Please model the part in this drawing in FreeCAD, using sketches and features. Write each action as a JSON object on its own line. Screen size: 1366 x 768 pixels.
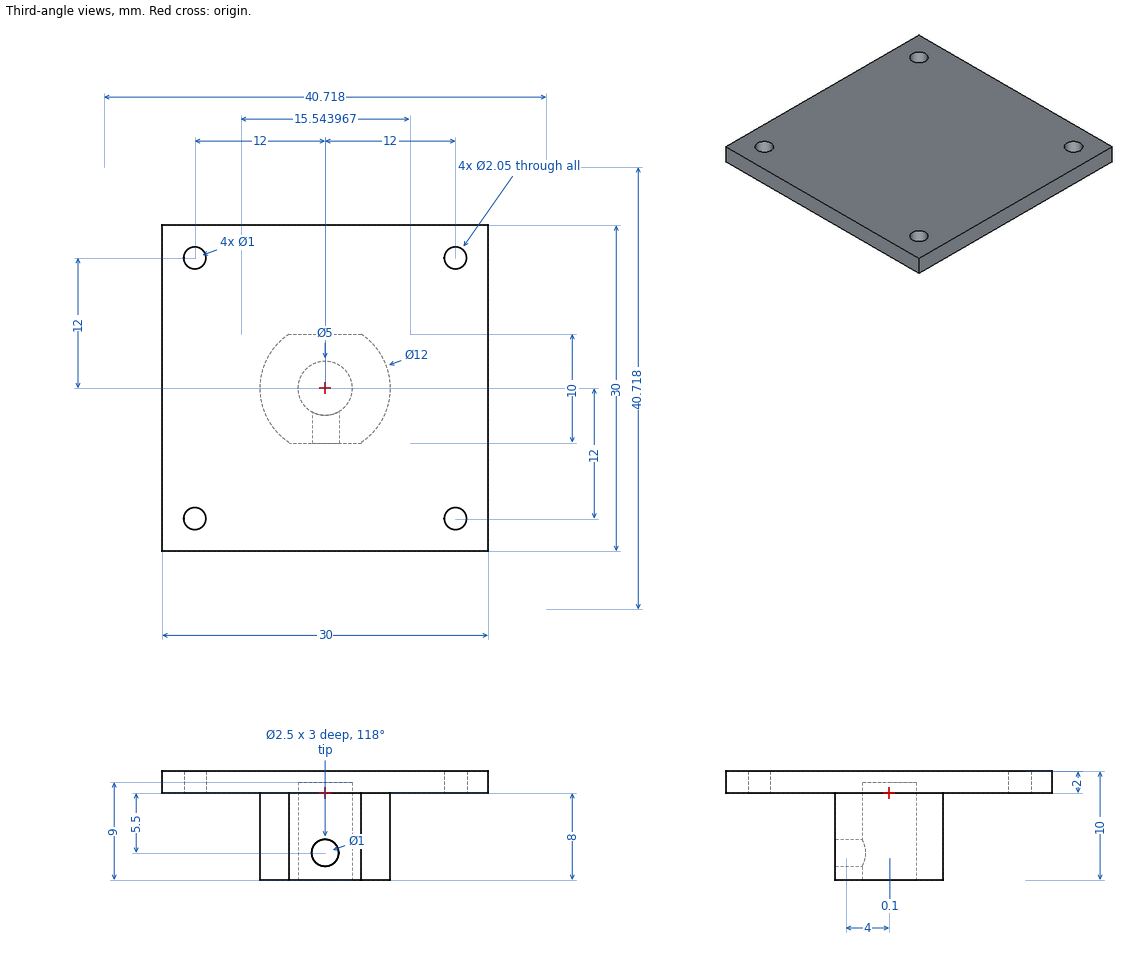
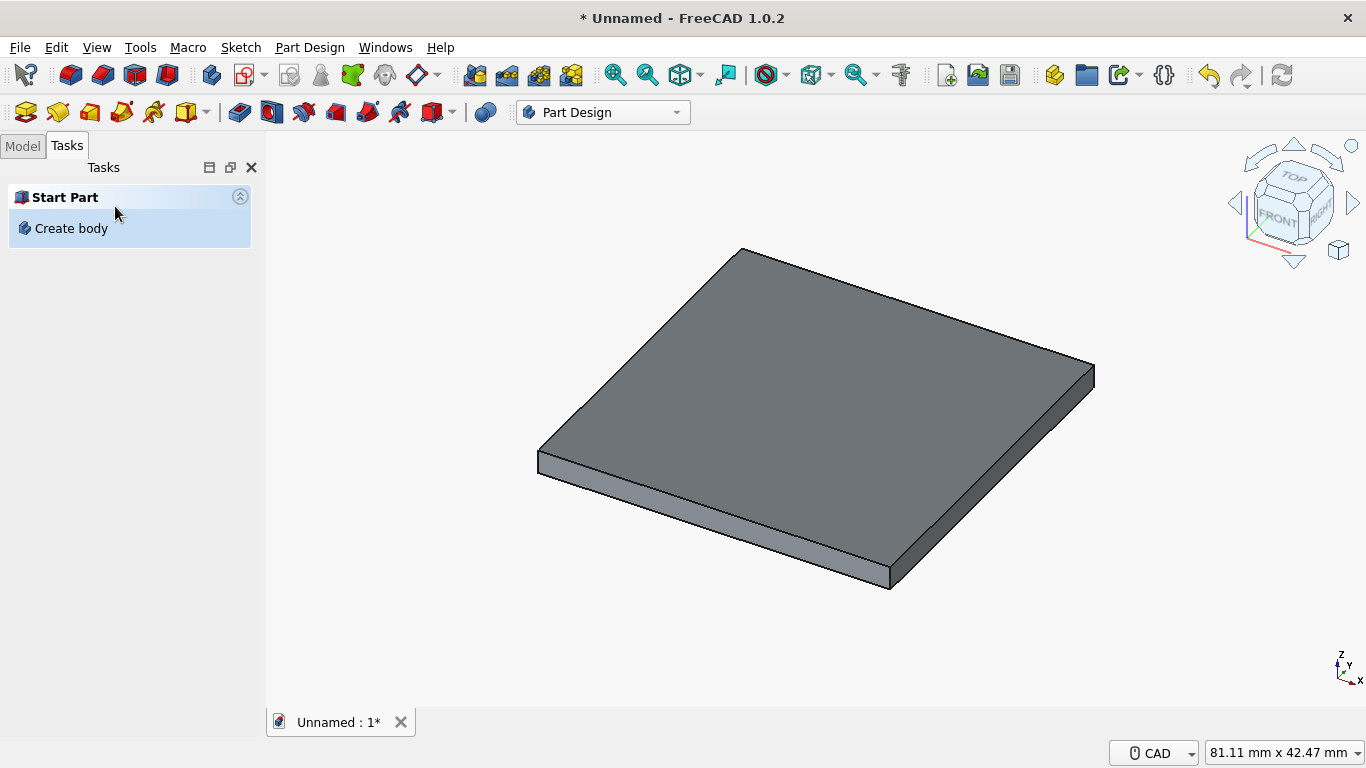
{"action": "key", "text": "5"}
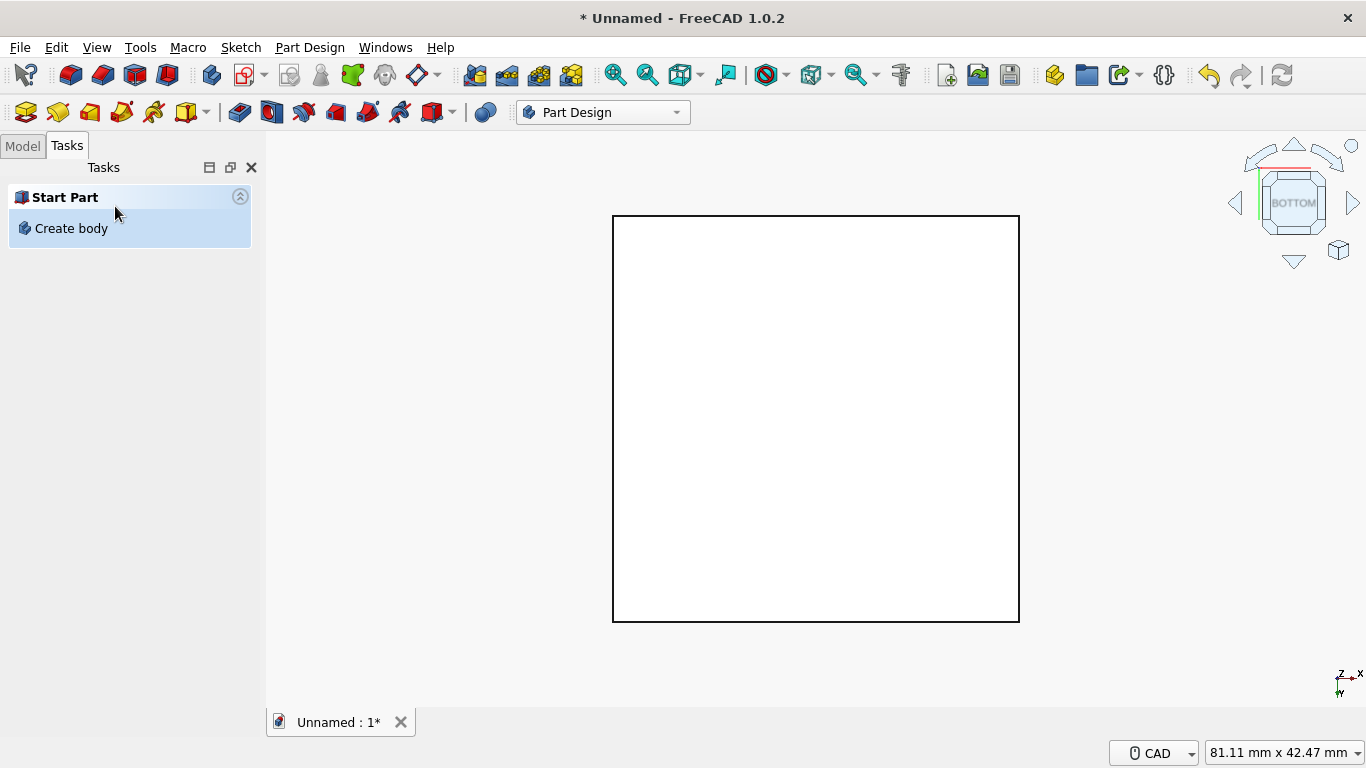
{"action": "left_click", "coordinate": [816, 418]}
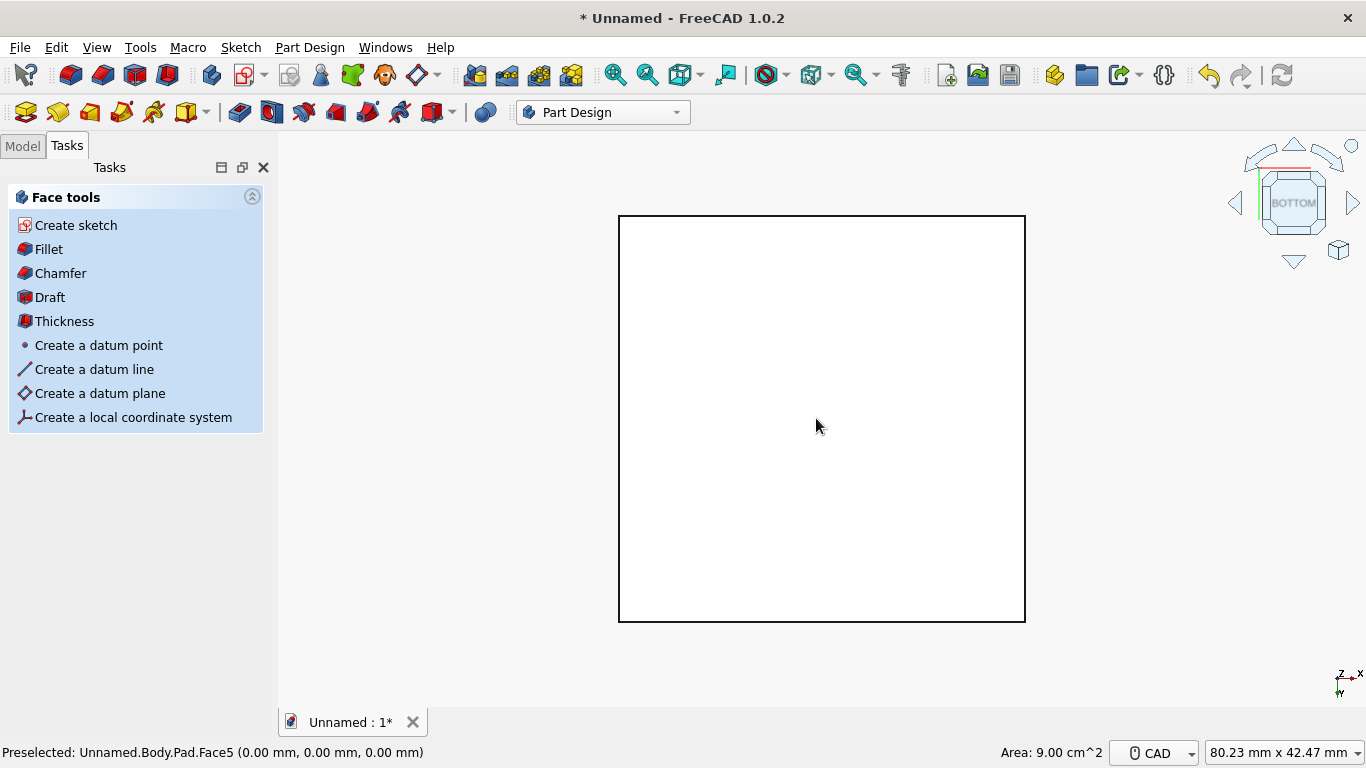
{"action": "left_click", "coordinate": [244, 76]}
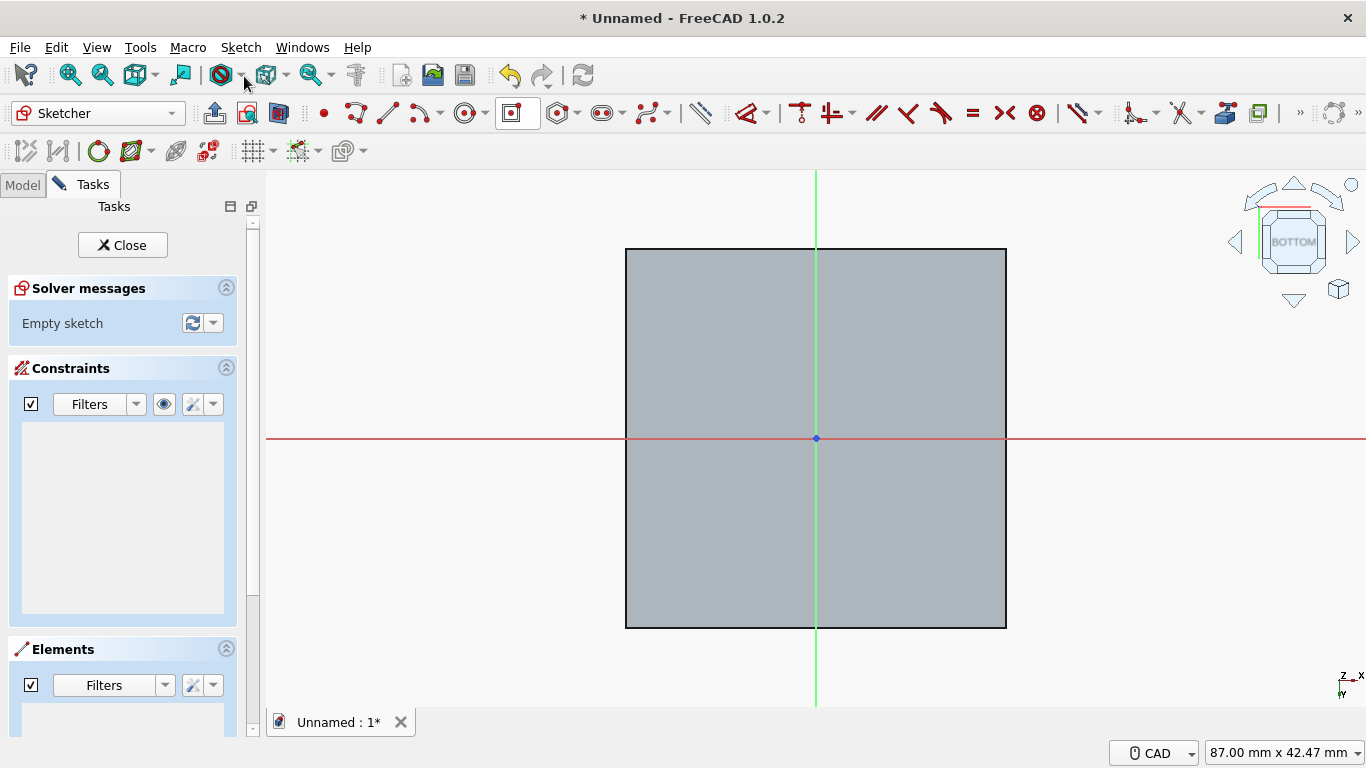
{"action": "scroll", "coordinate": [872, 438], "scroll_direction": "up", "scroll_amount": 4}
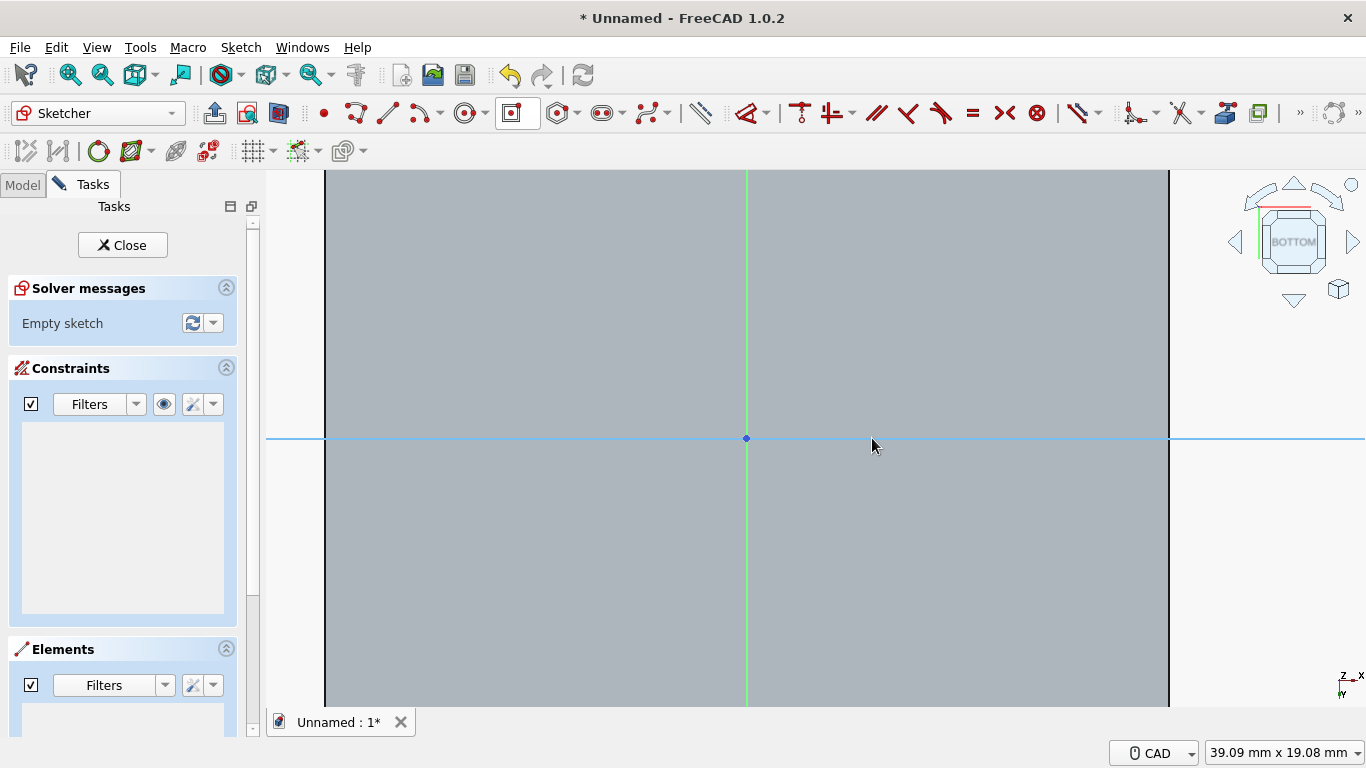
{"action": "left_click", "coordinate": [466, 114]}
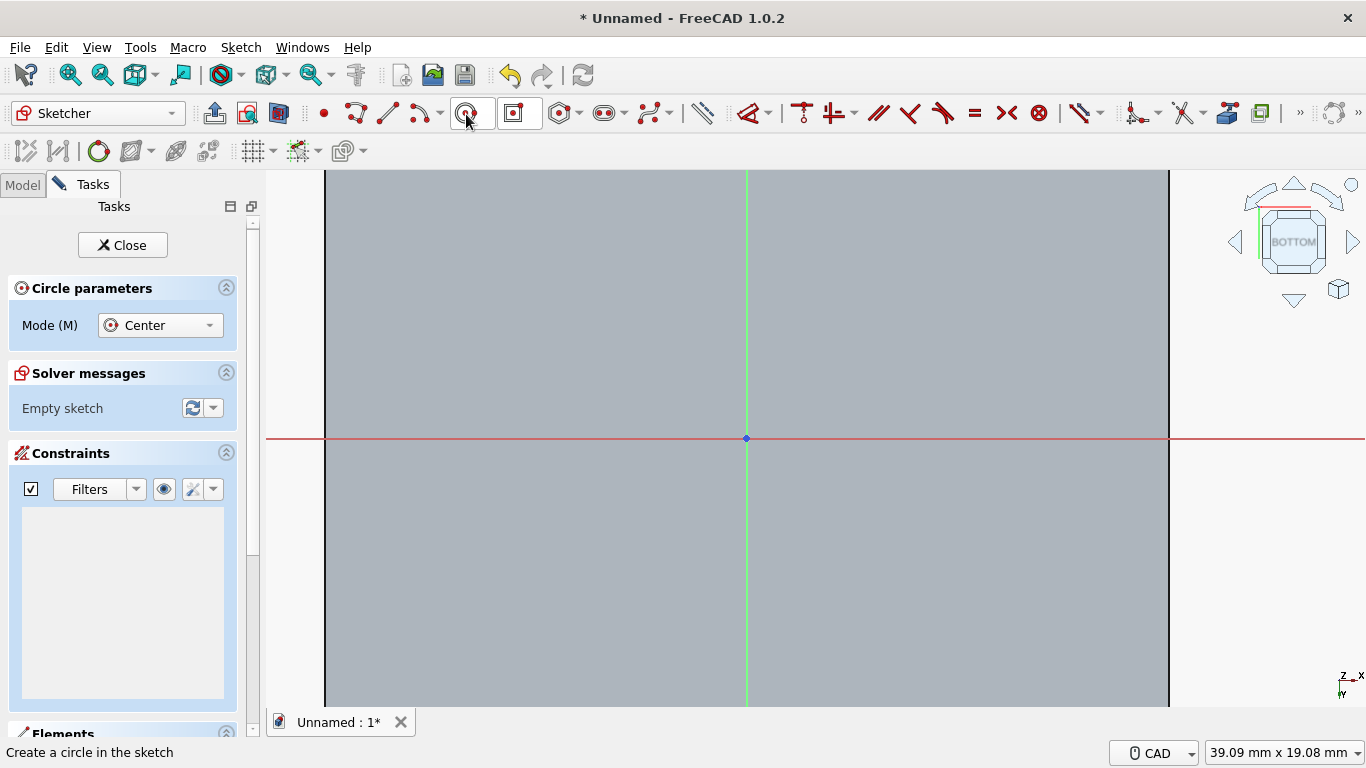
{"action": "left_click", "coordinate": [747, 438]}
{"action": "left_click", "coordinate": [866, 319]}
{"action": "key", "text": "Escape"}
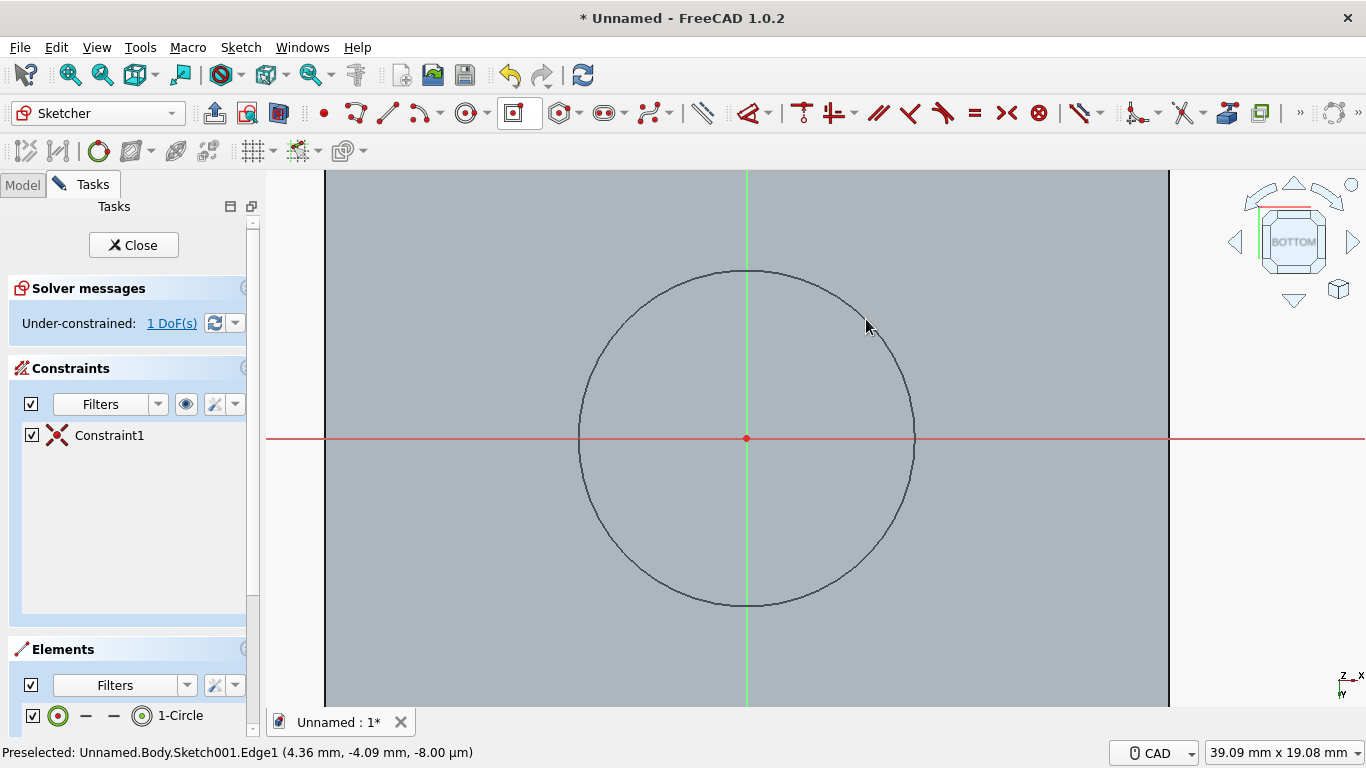
{"action": "left_click", "coordinate": [748, 114]}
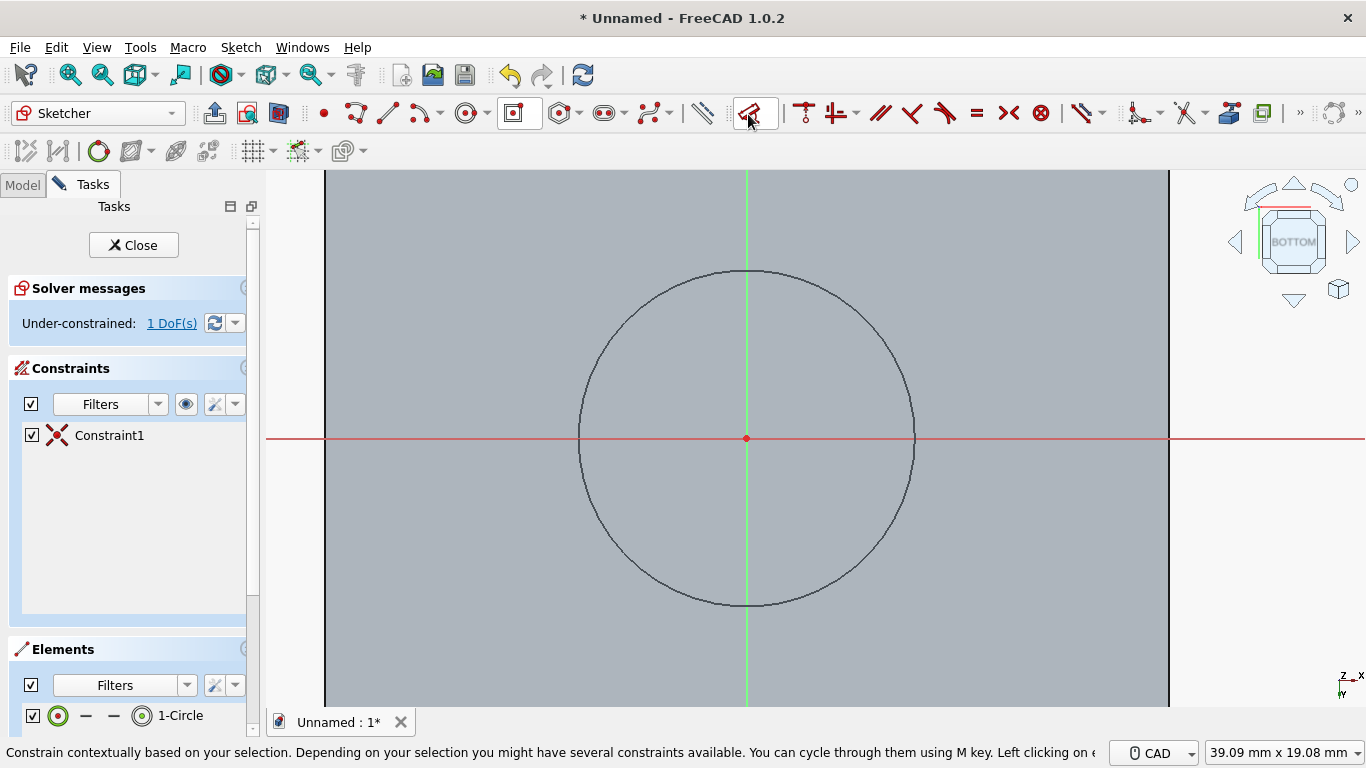
{"action": "left_click", "coordinate": [865, 319]}
{"action": "left_click", "coordinate": [888, 296]}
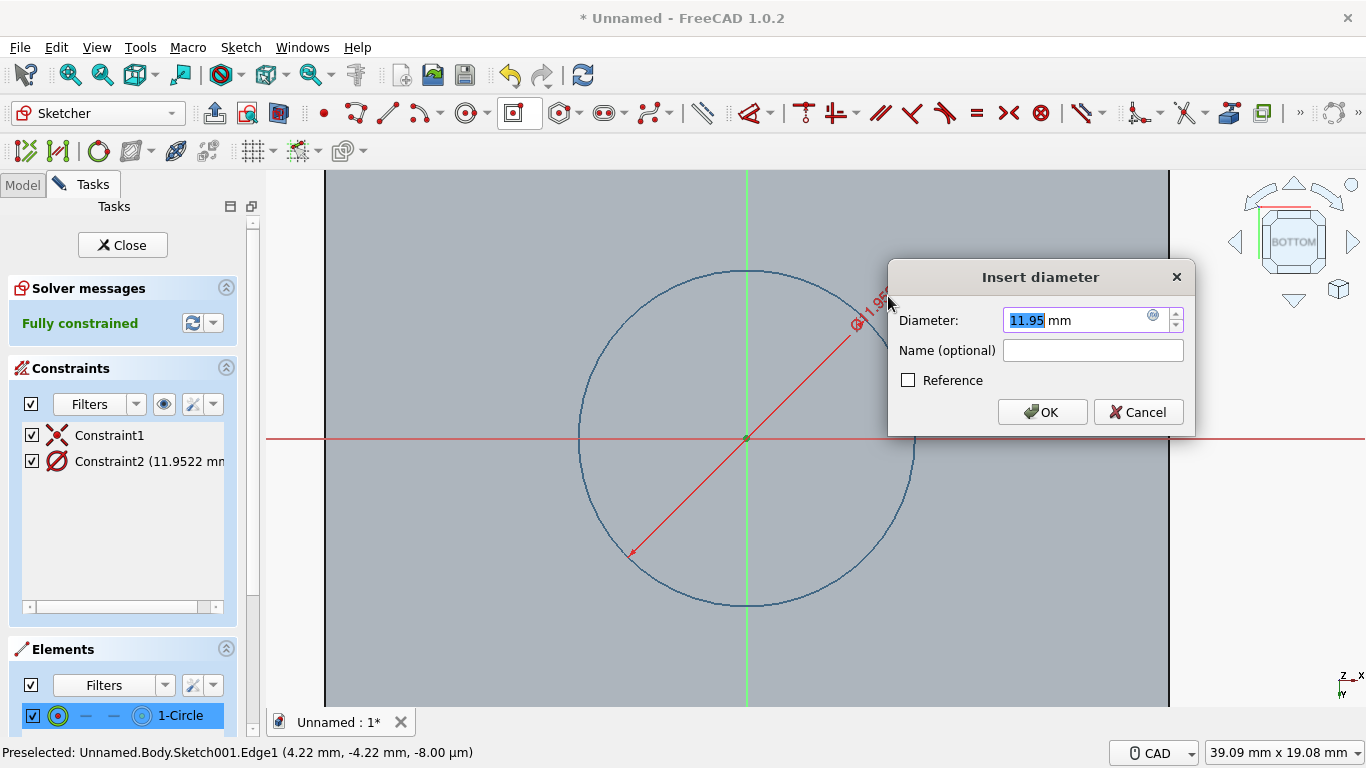
{"action": "type", "text": "12"}
{"action": "key", "text": "Return"}
{"action": "key", "text": "Escape"}